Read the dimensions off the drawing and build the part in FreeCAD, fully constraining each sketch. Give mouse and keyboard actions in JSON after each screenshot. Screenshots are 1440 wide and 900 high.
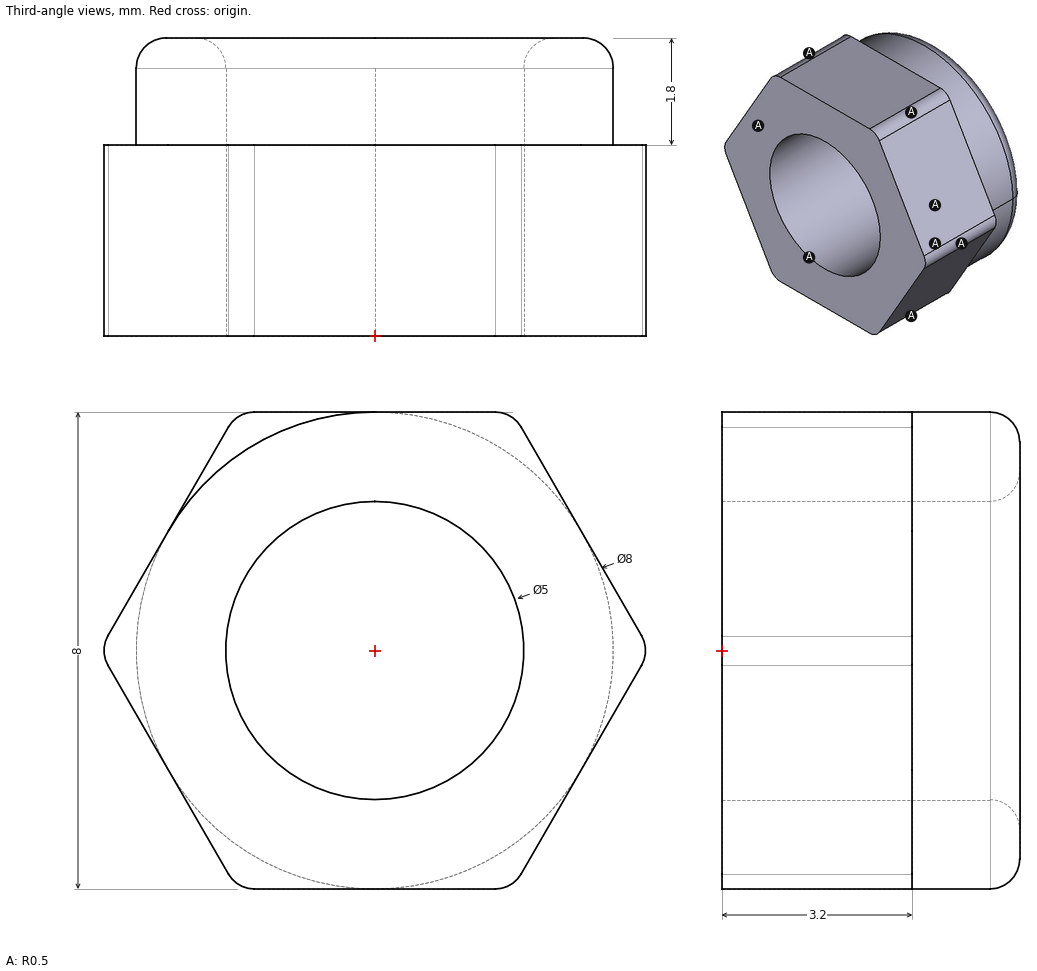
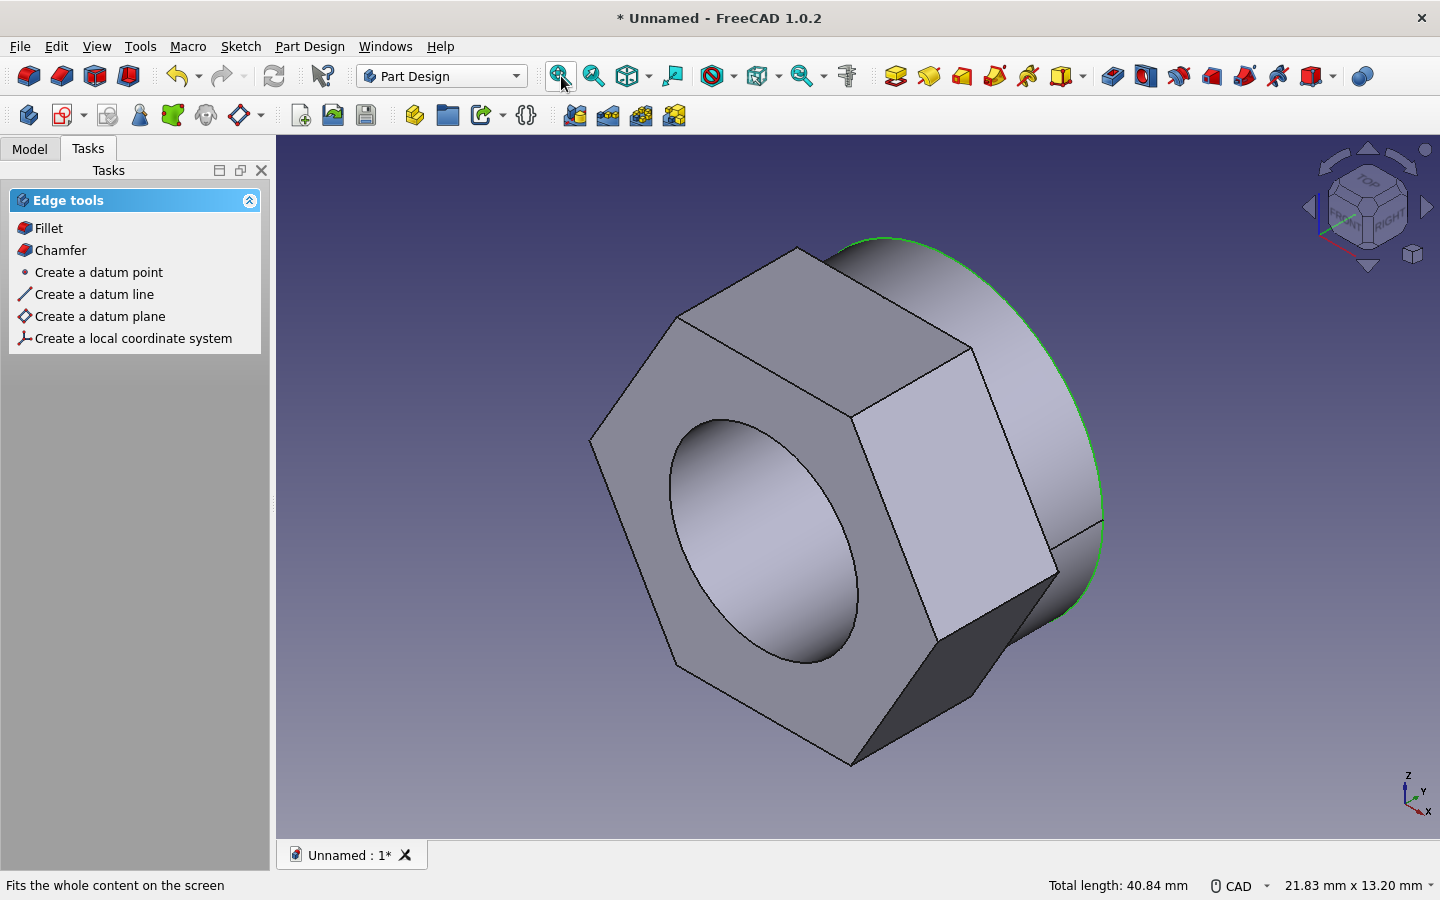
{"action": "left_click", "coordinate": [911, 382], "text": "ctrl"}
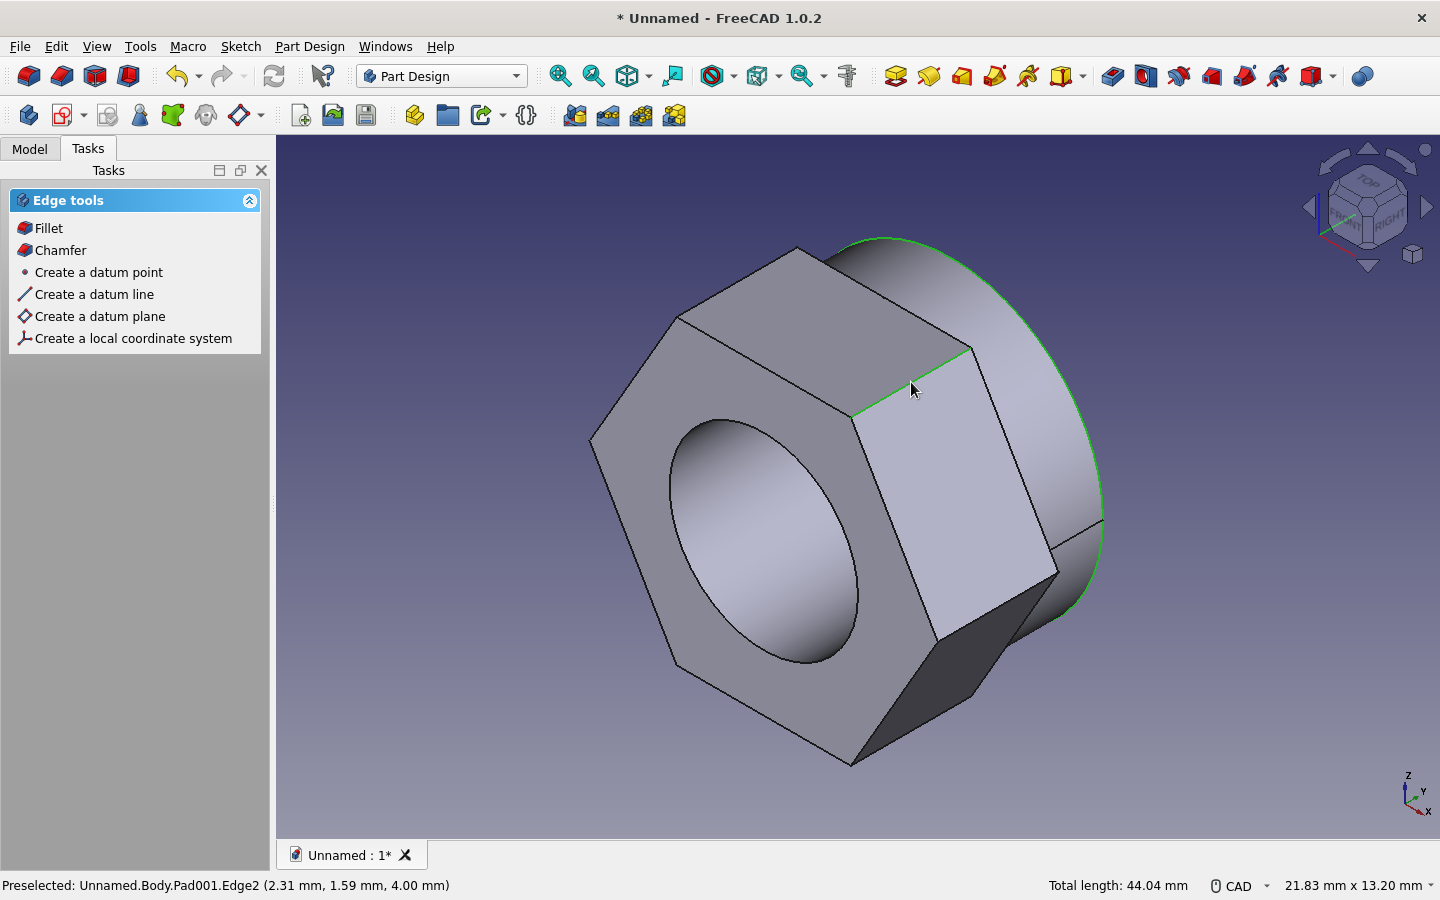
{"action": "key", "text": "2"}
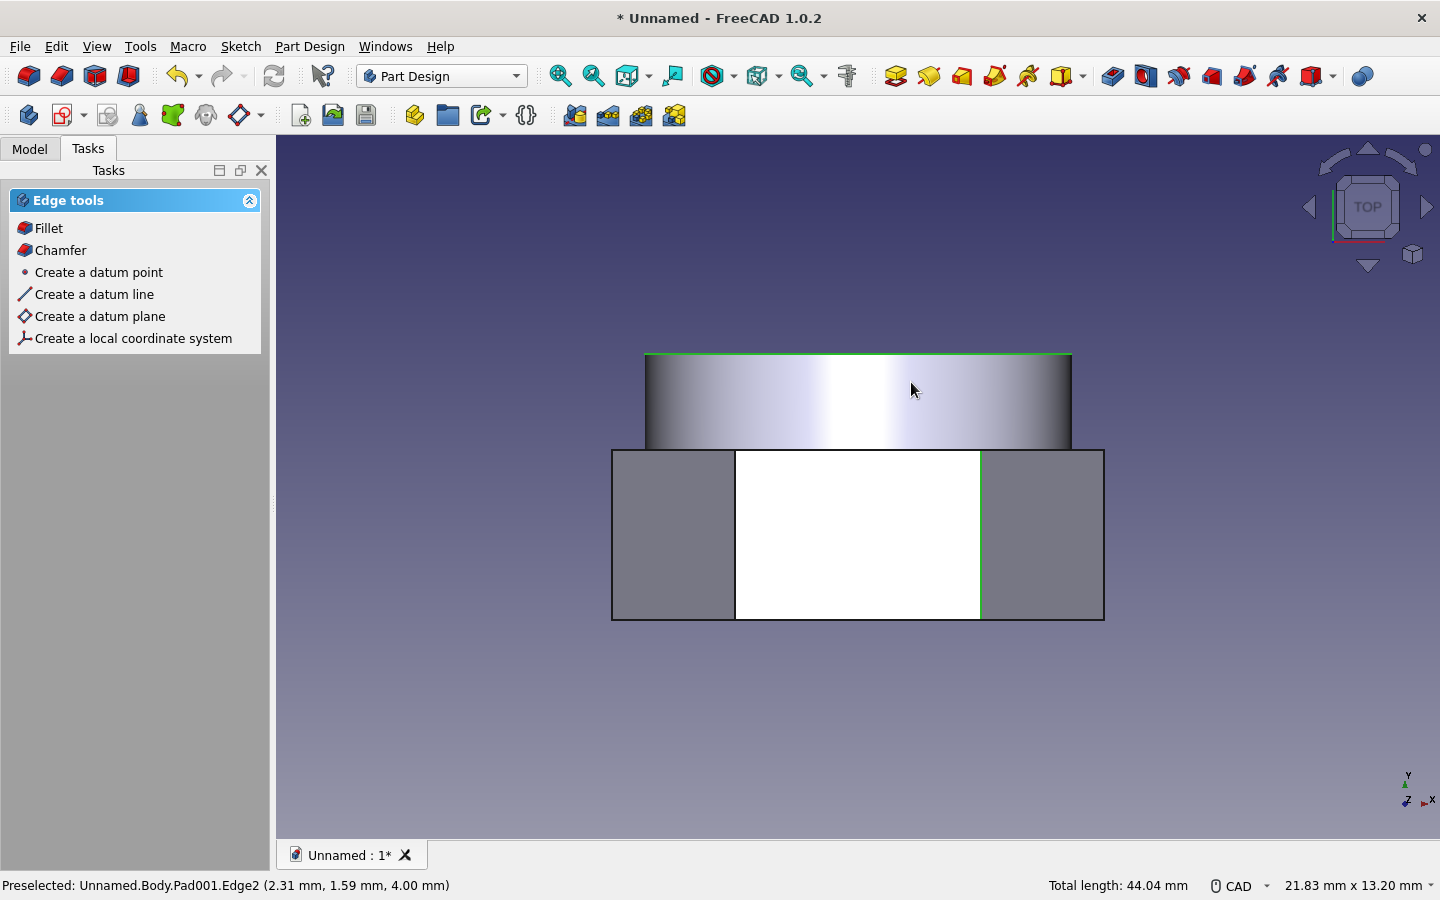
{"action": "left_click", "coordinate": [561, 76]}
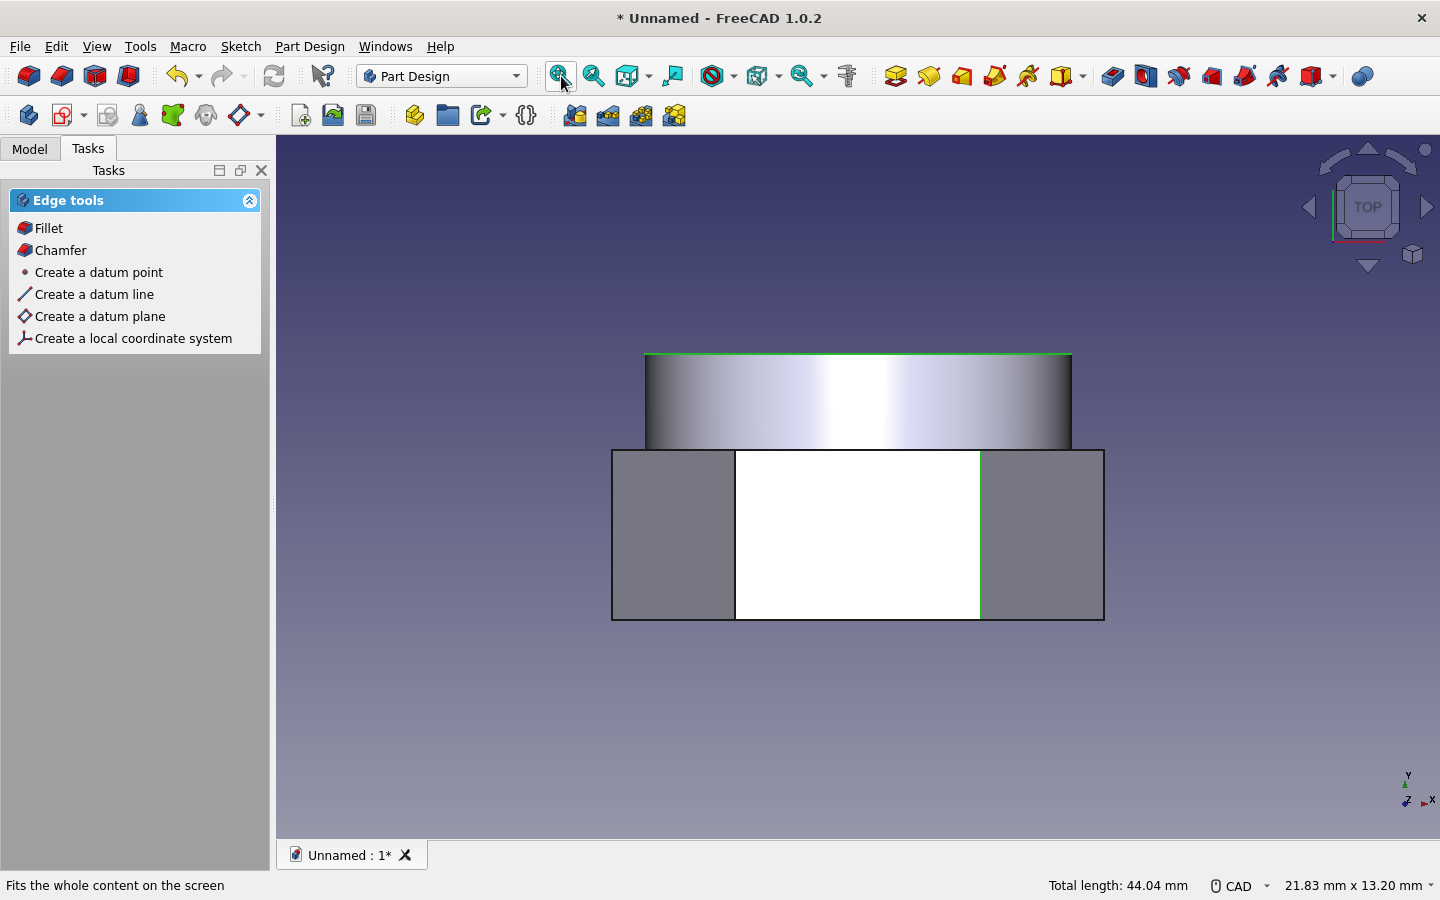
{"action": "left_click", "coordinate": [735, 534], "text": "ctrl"}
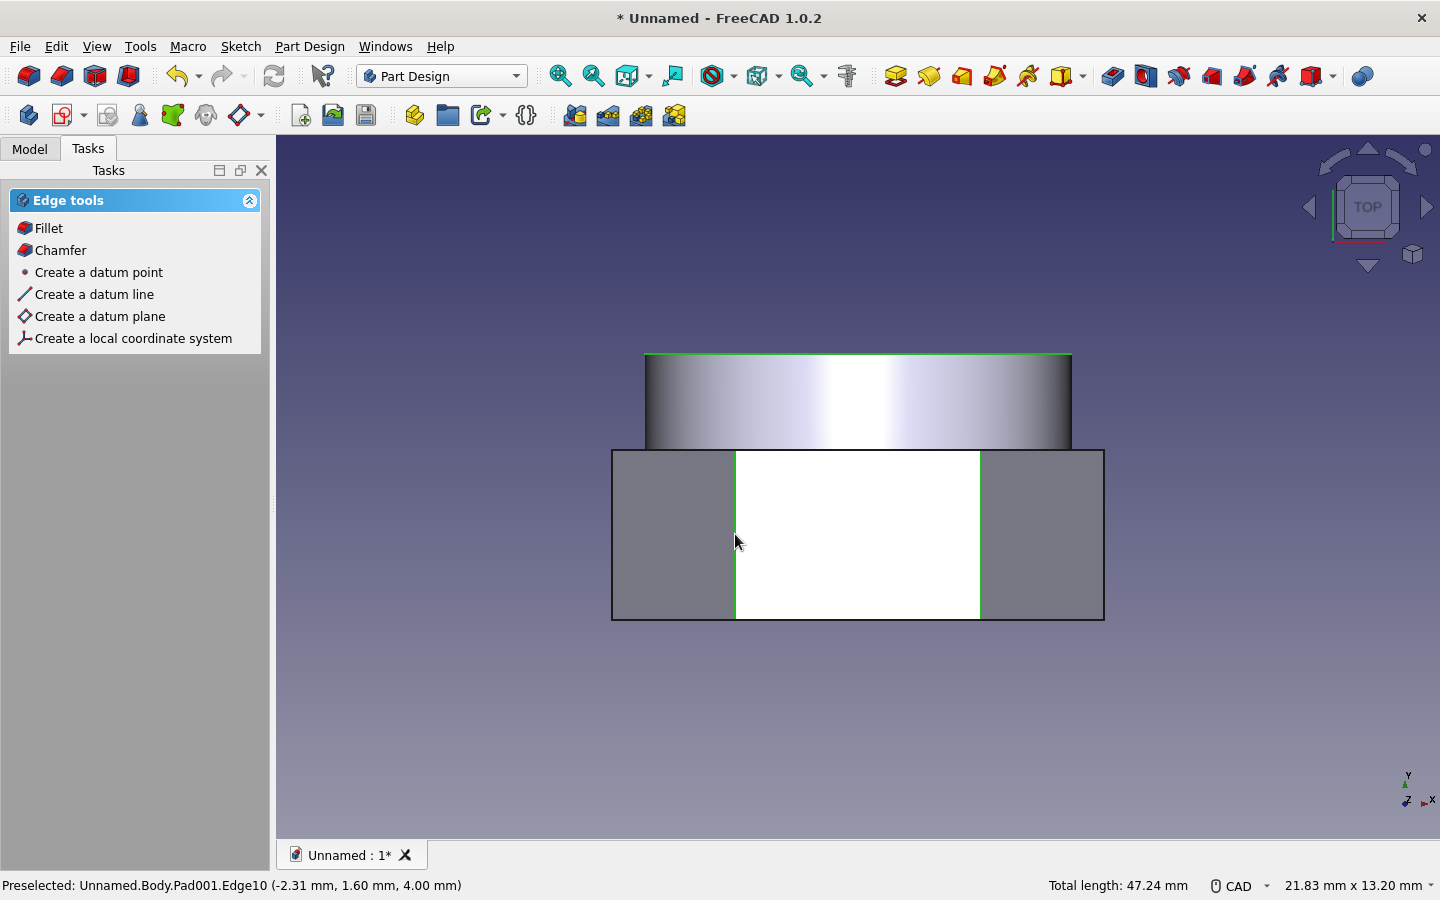
{"action": "key", "text": "1"}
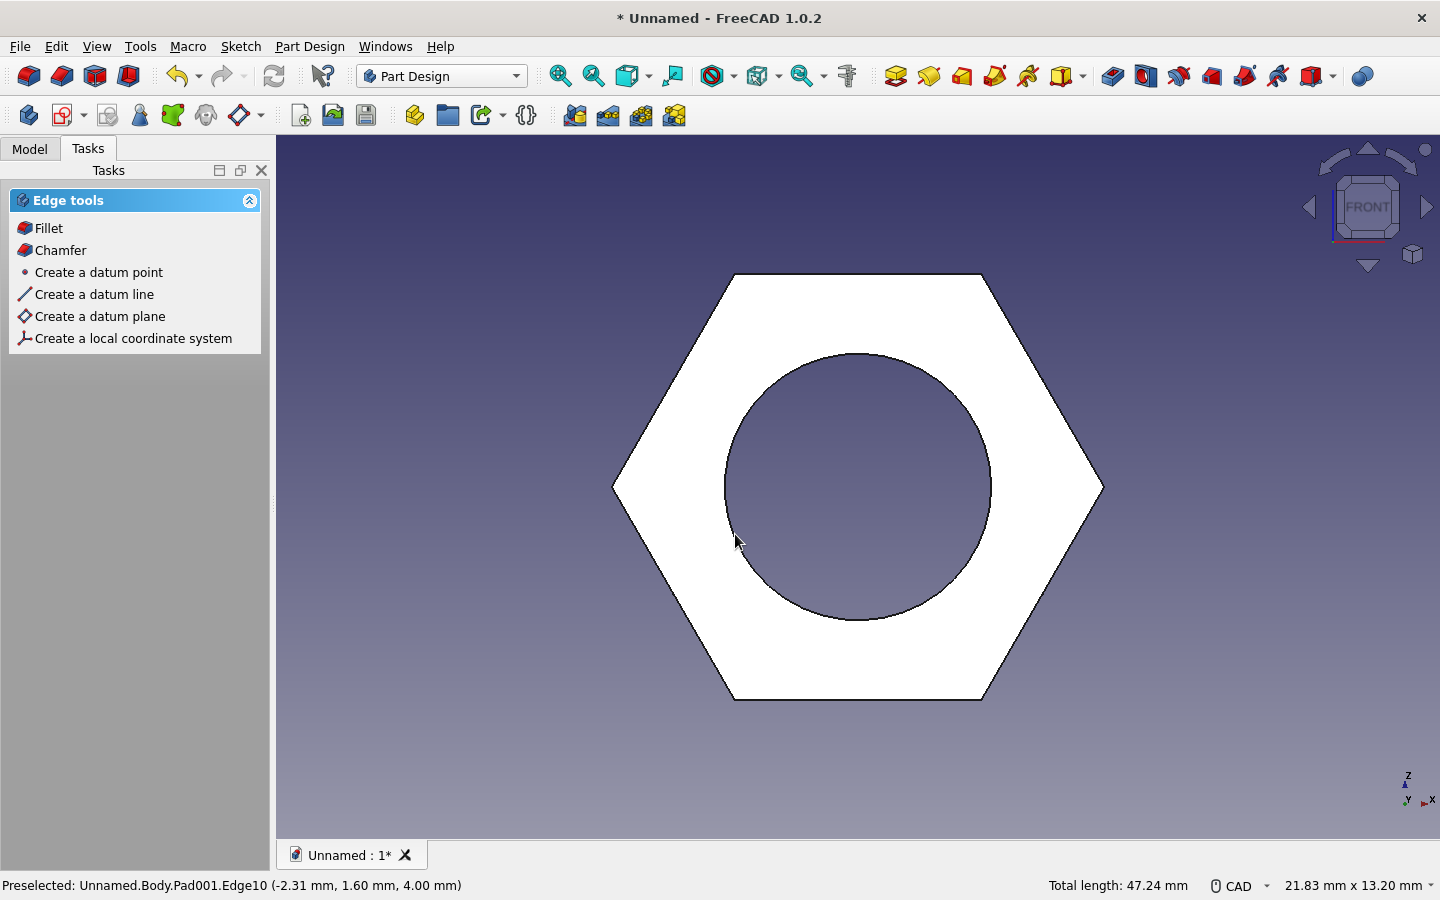
{"action": "key", "text": "3"}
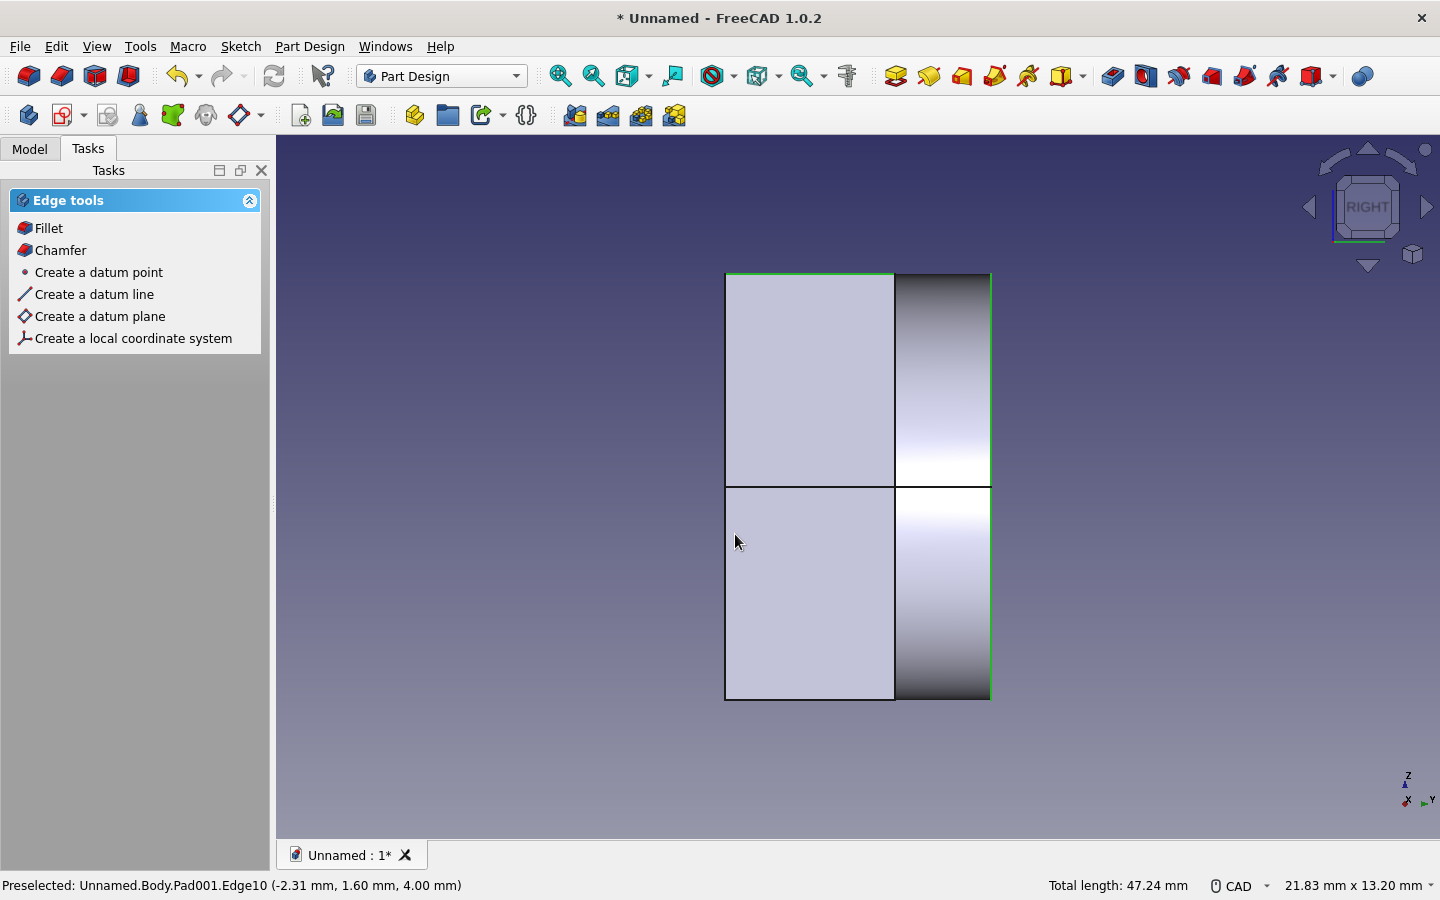
{"action": "left_click", "coordinate": [810, 486], "text": "ctrl"}